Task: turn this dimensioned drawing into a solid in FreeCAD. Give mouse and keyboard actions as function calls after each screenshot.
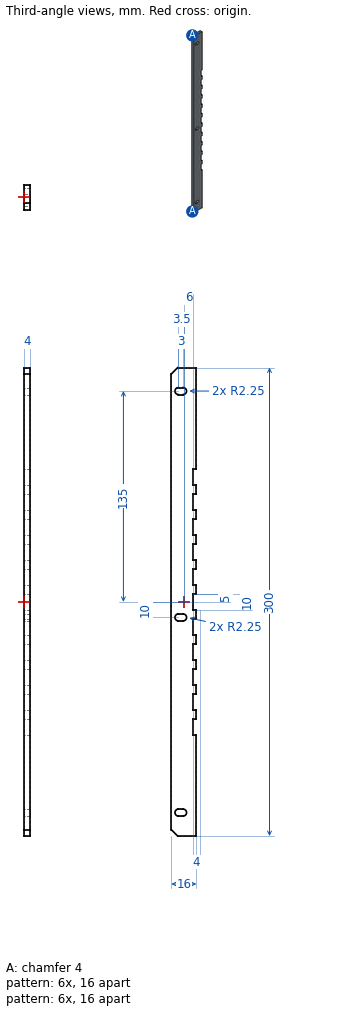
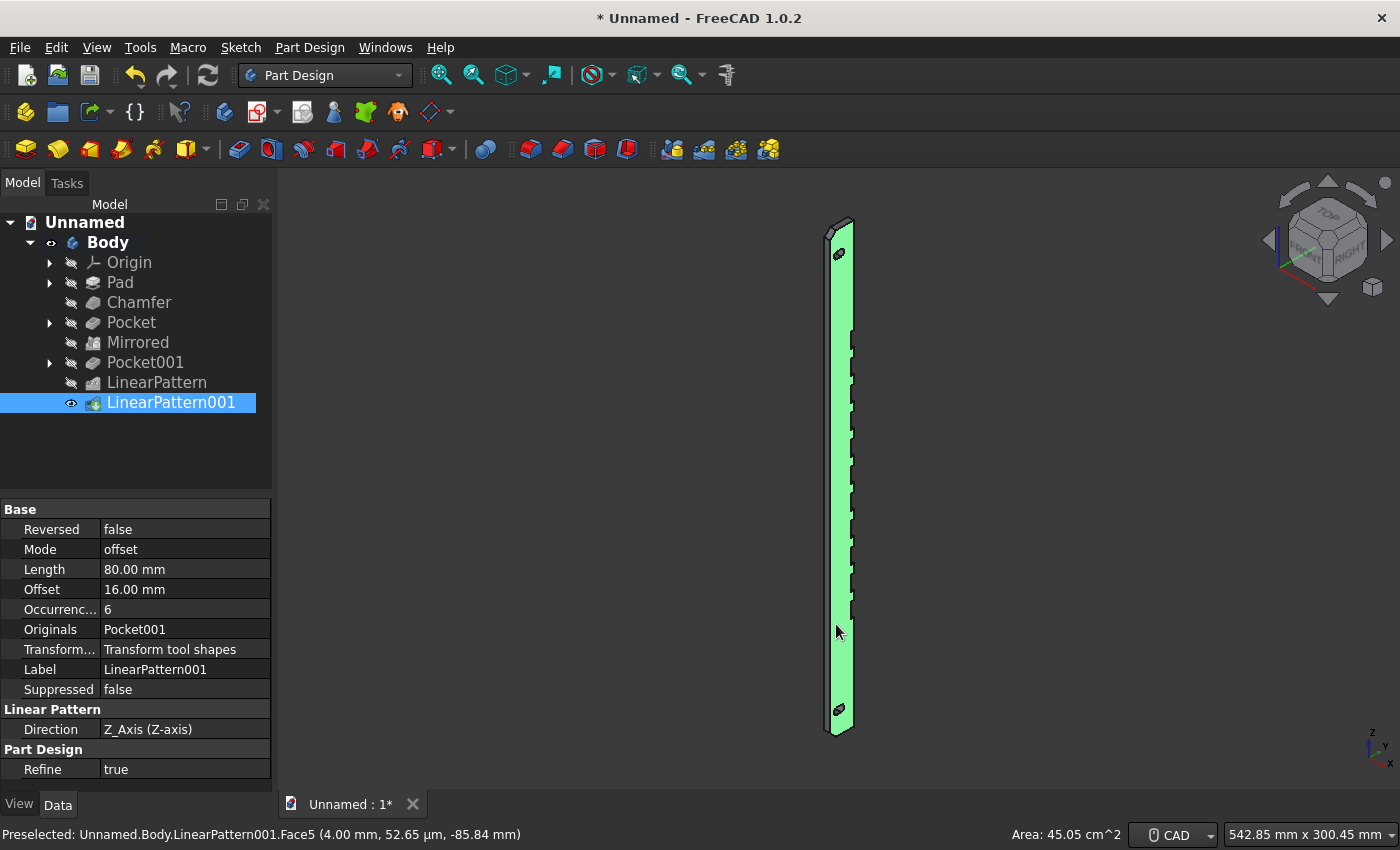
click(258, 112)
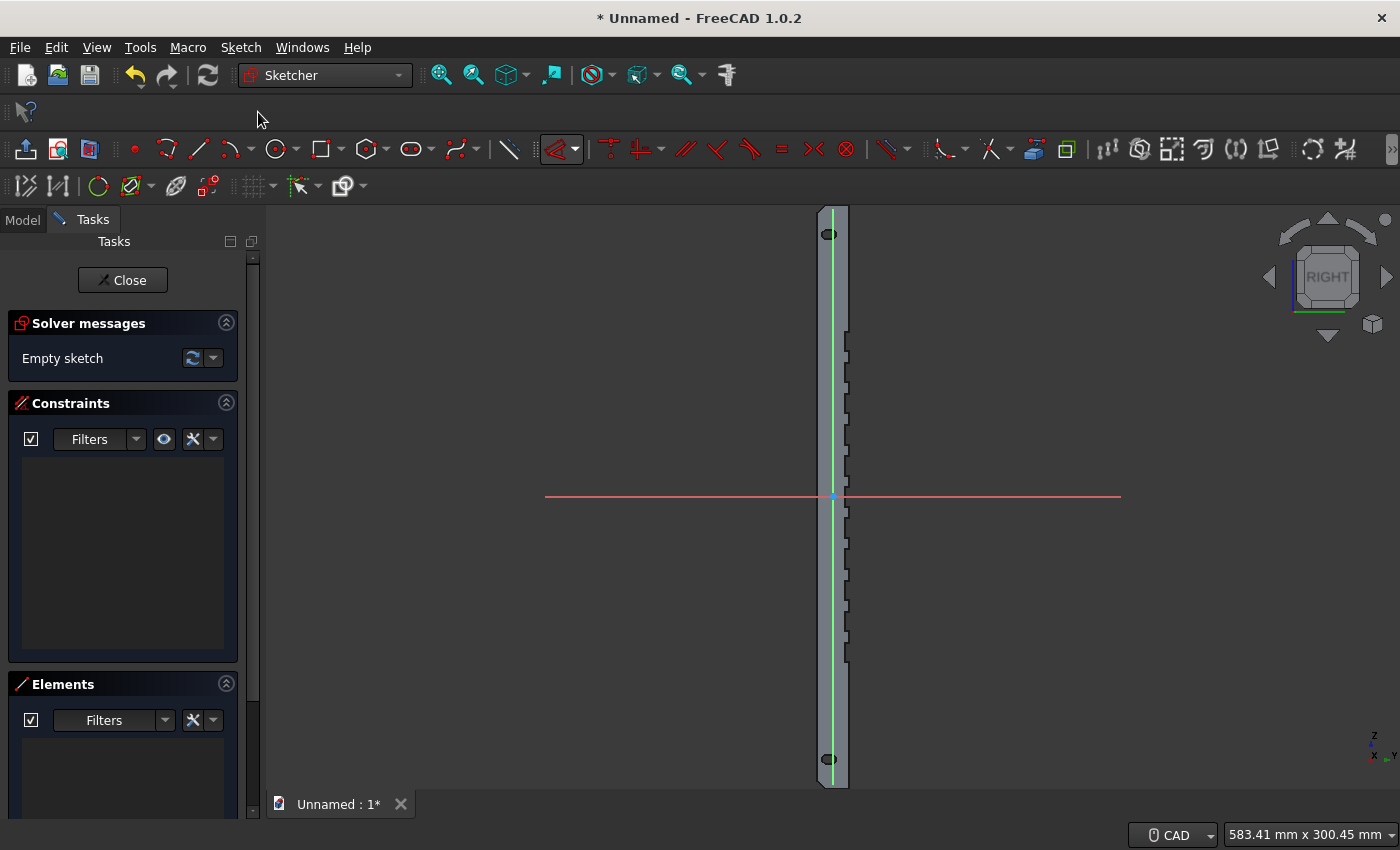
scroll(833, 510, up, 14)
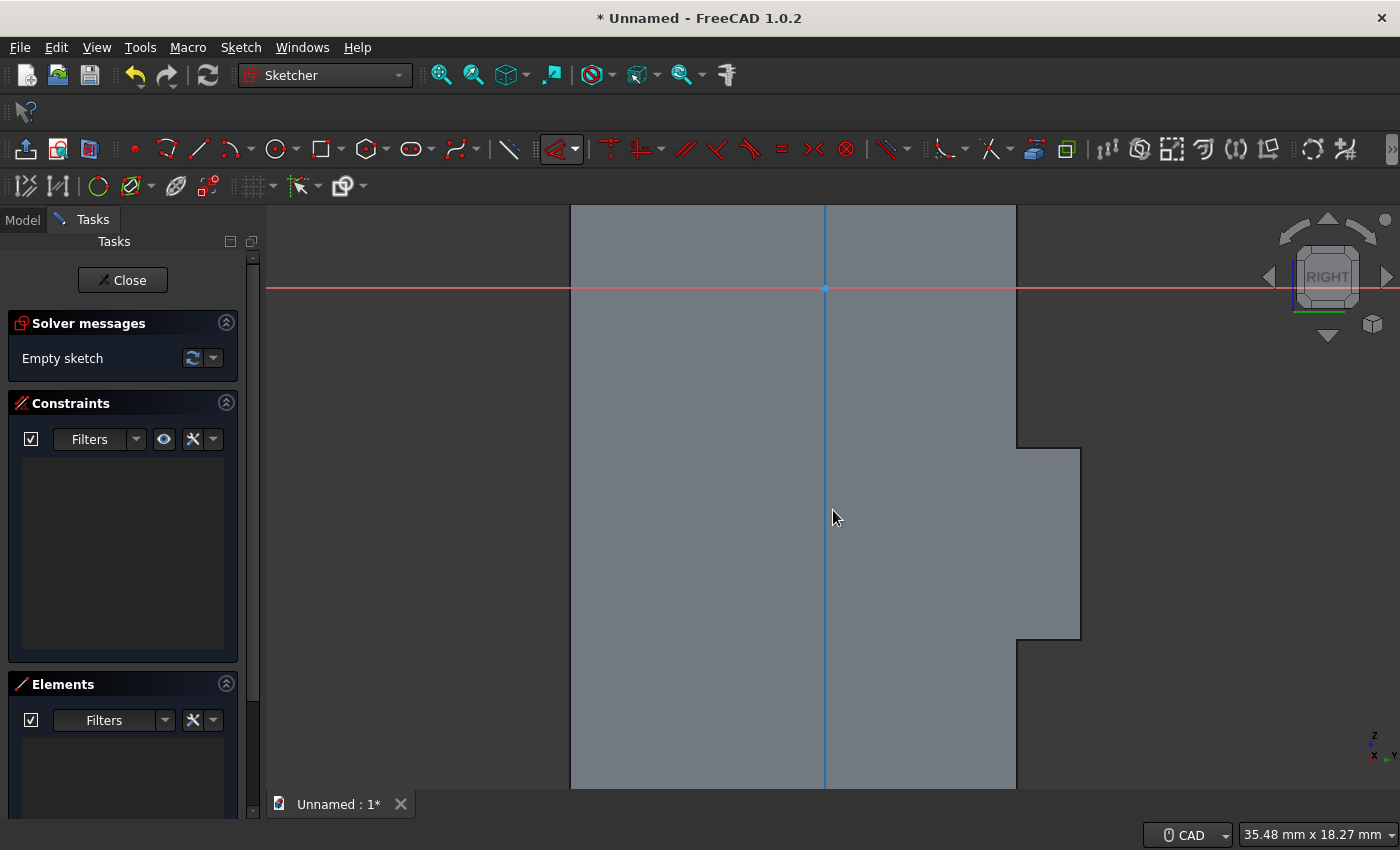
click(412, 150)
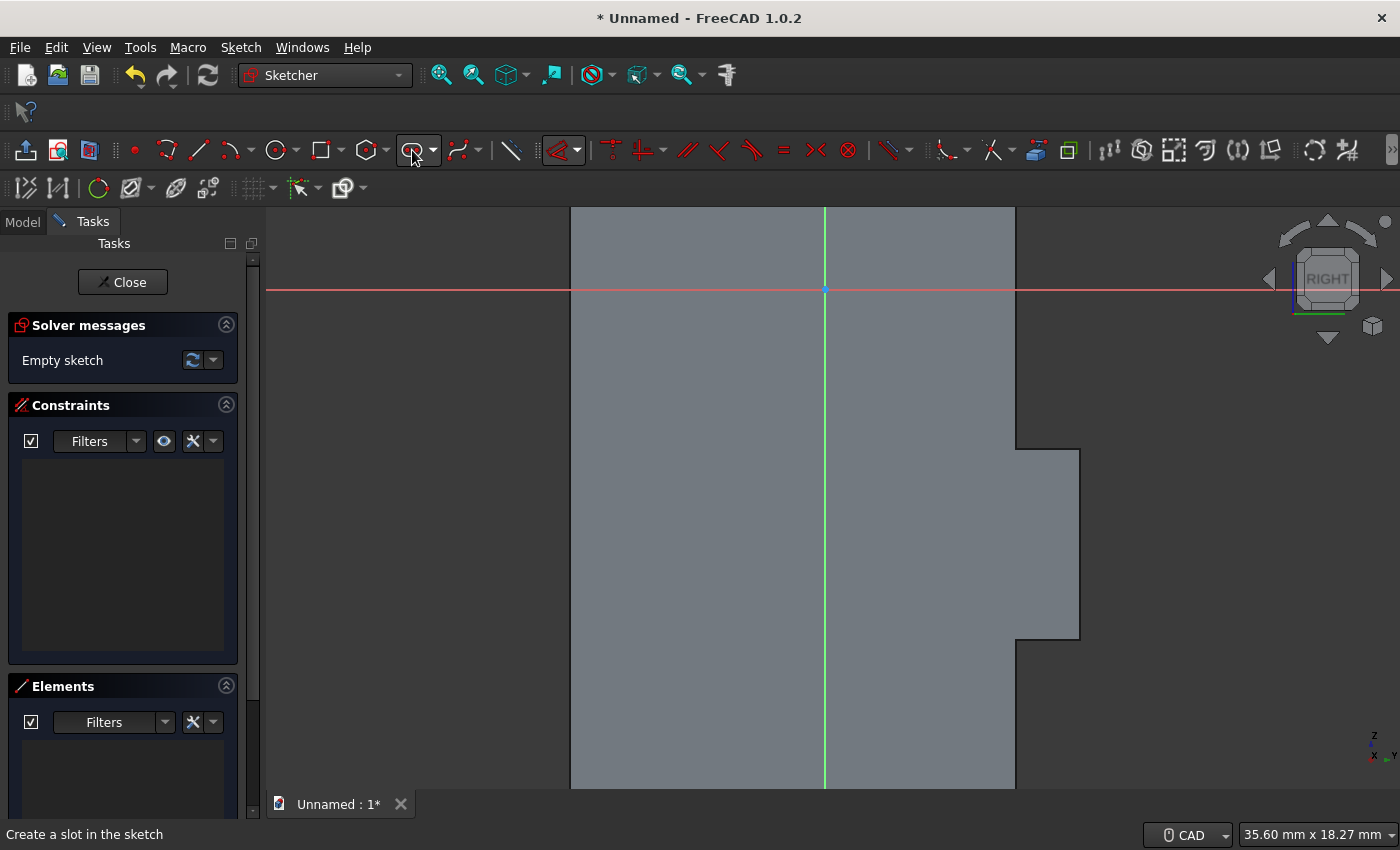
click(714, 608)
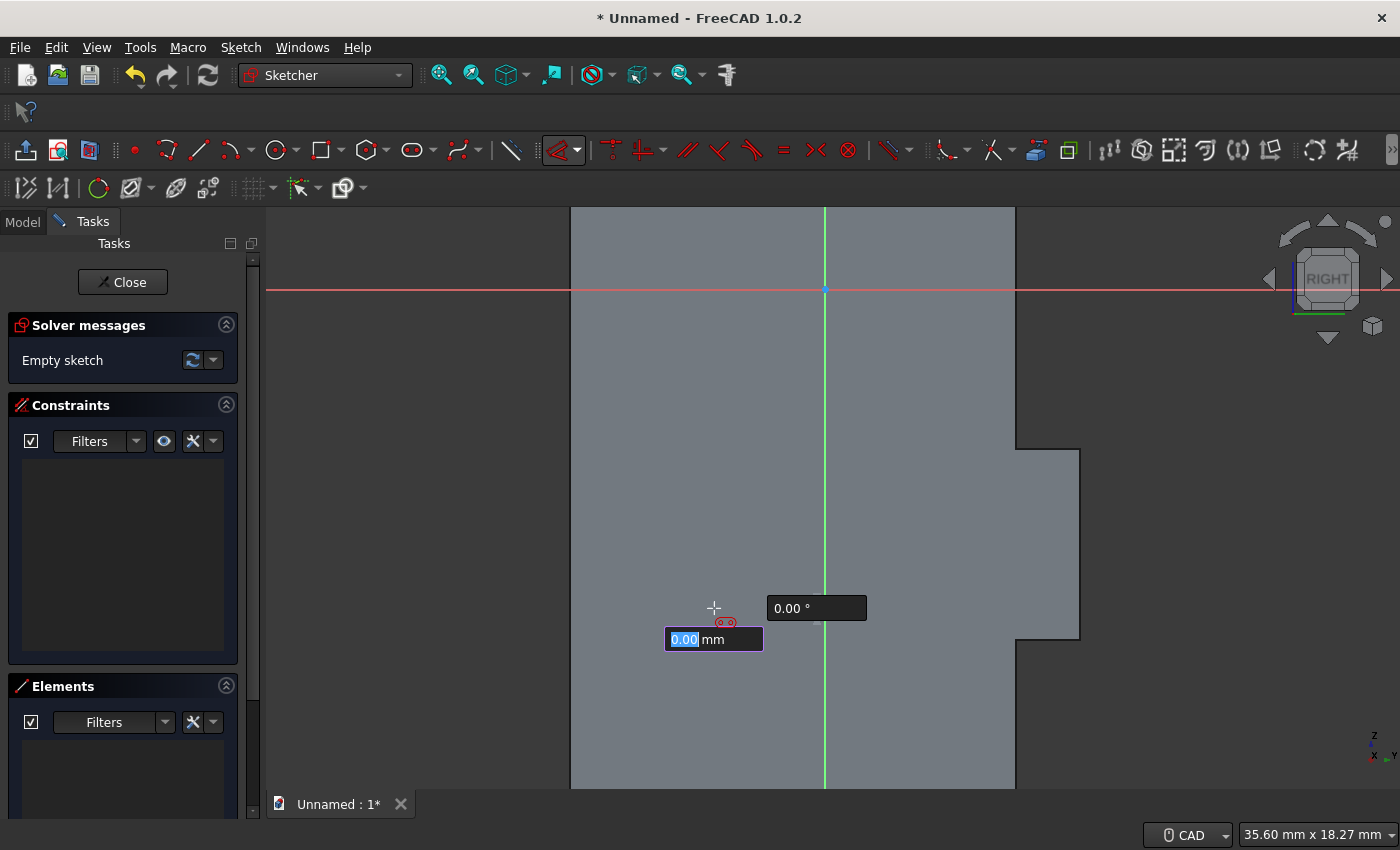
click(809, 608)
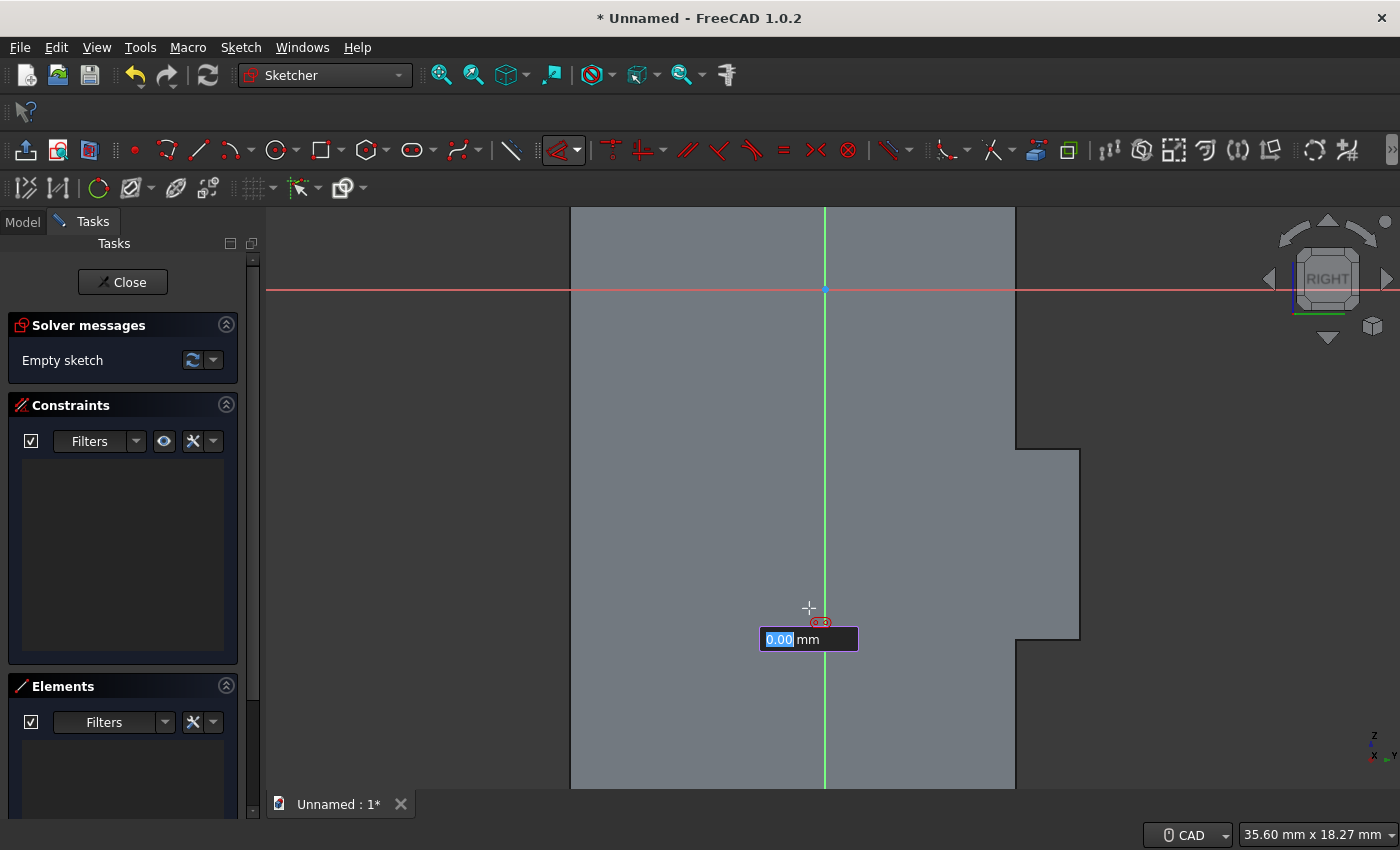
click(762, 680)
key(Escape)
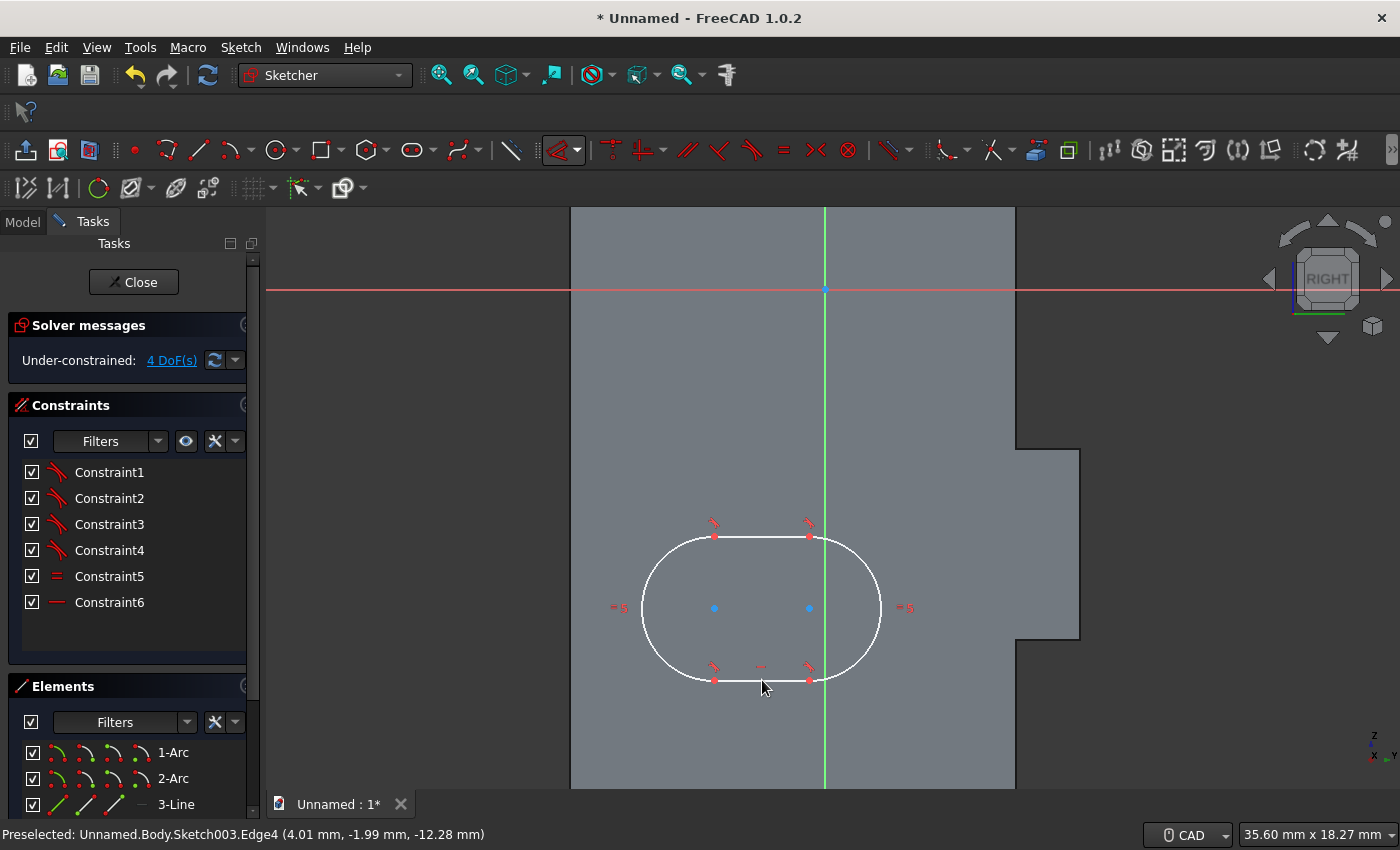
click(656, 567)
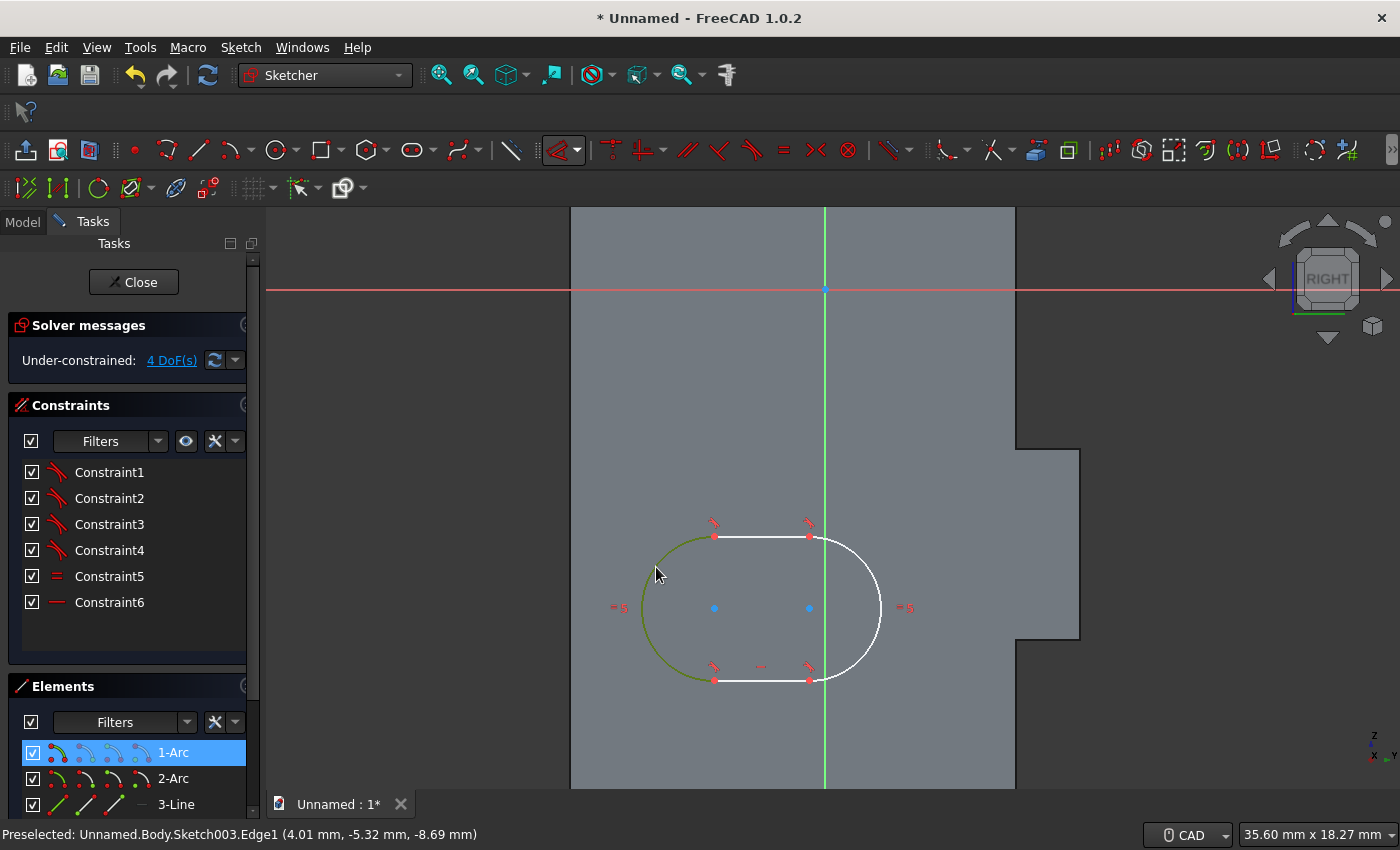
key(k)
key(r)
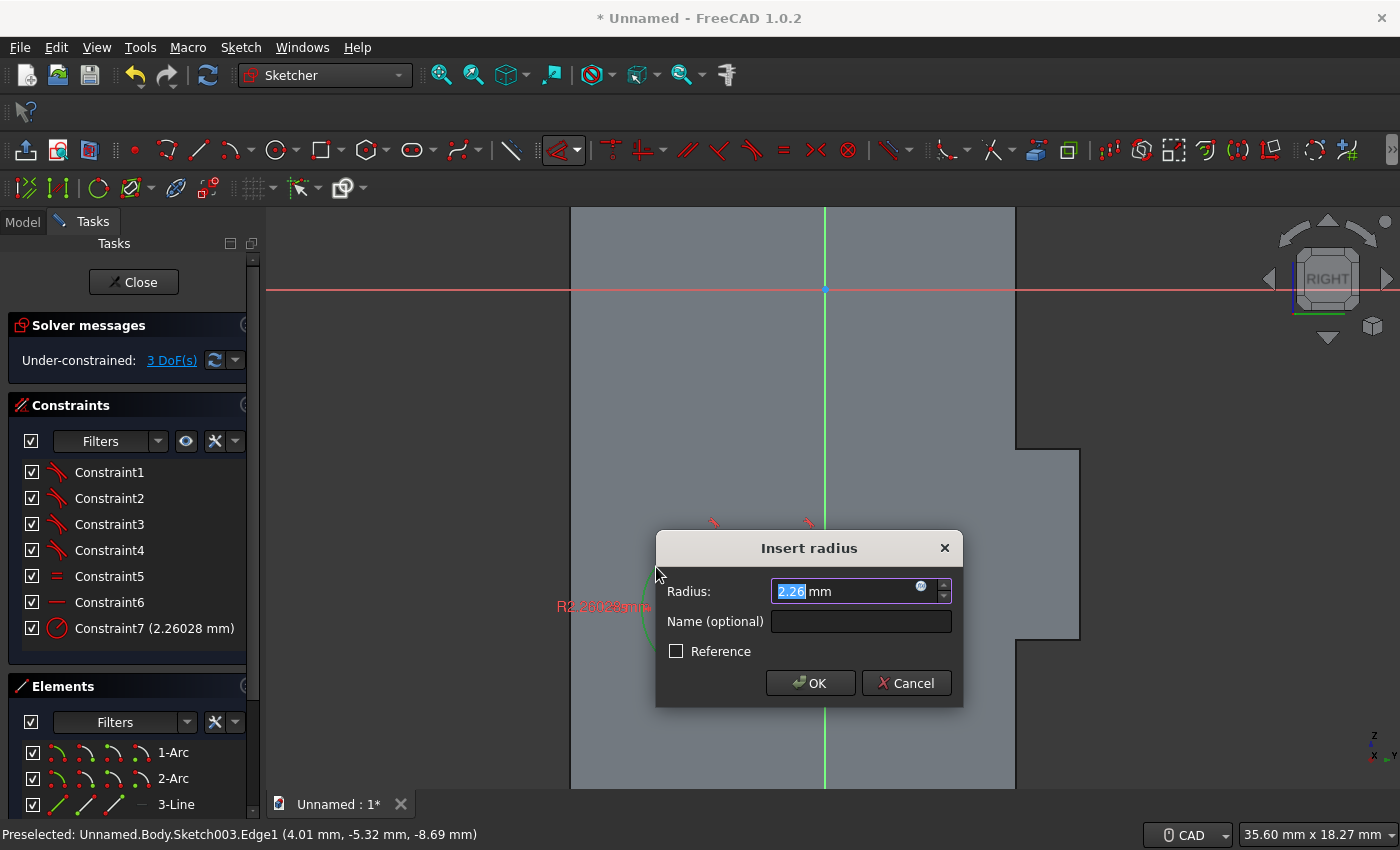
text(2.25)
key(Return)